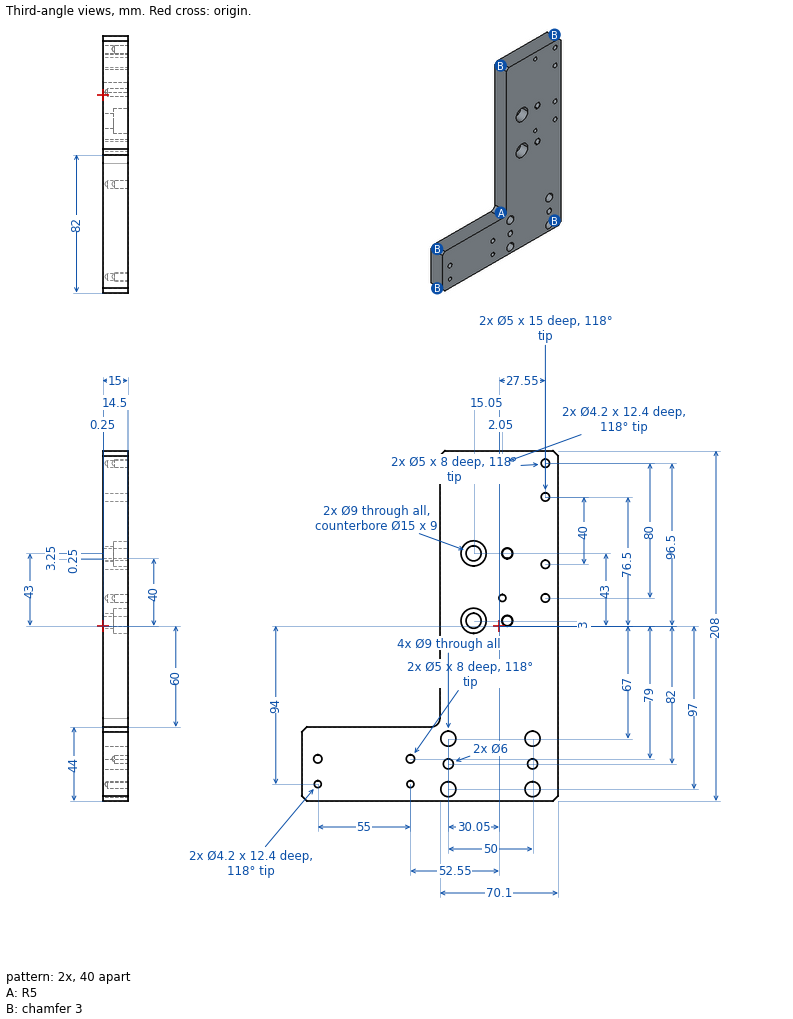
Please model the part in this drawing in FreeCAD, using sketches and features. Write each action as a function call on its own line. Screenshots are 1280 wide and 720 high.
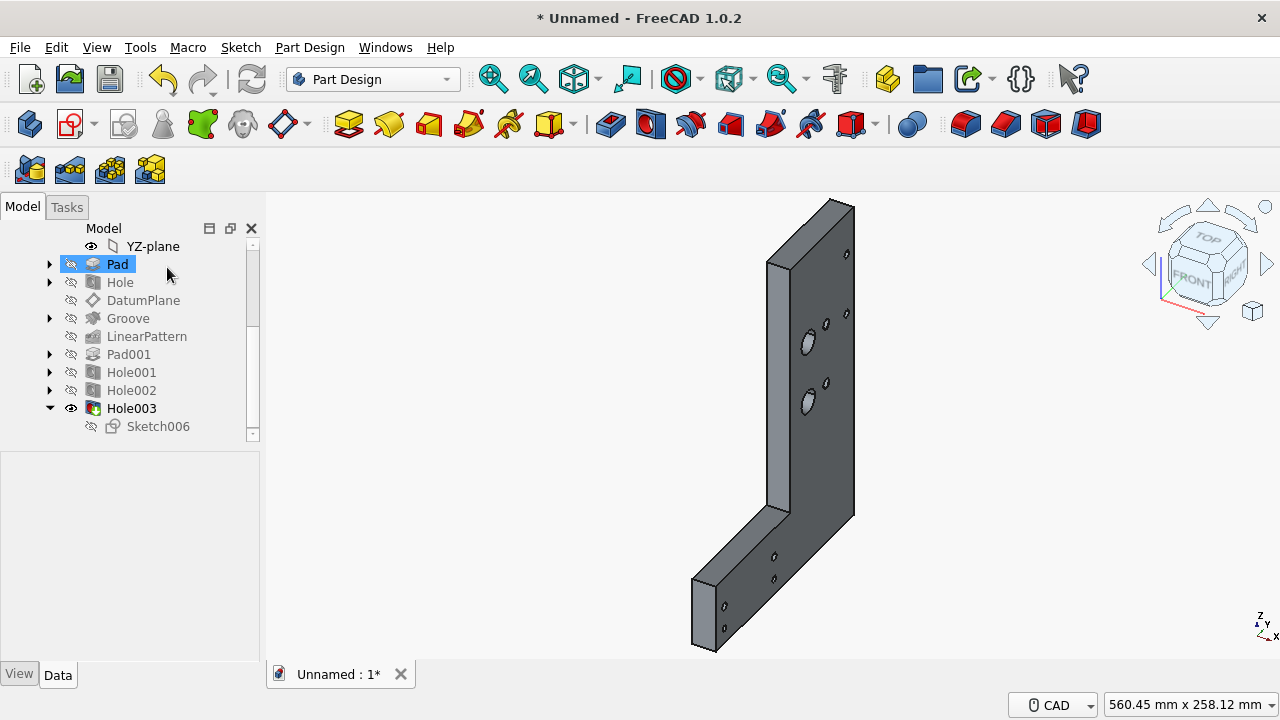
click(824, 477)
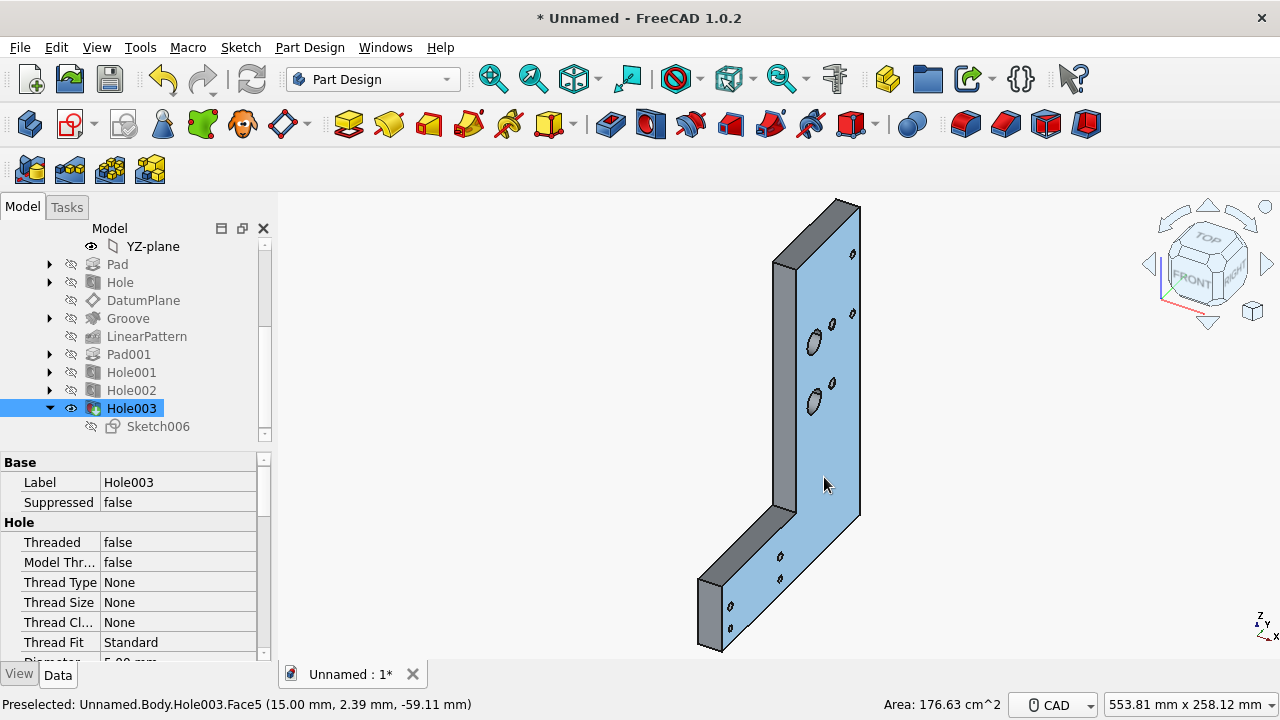
click(70, 124)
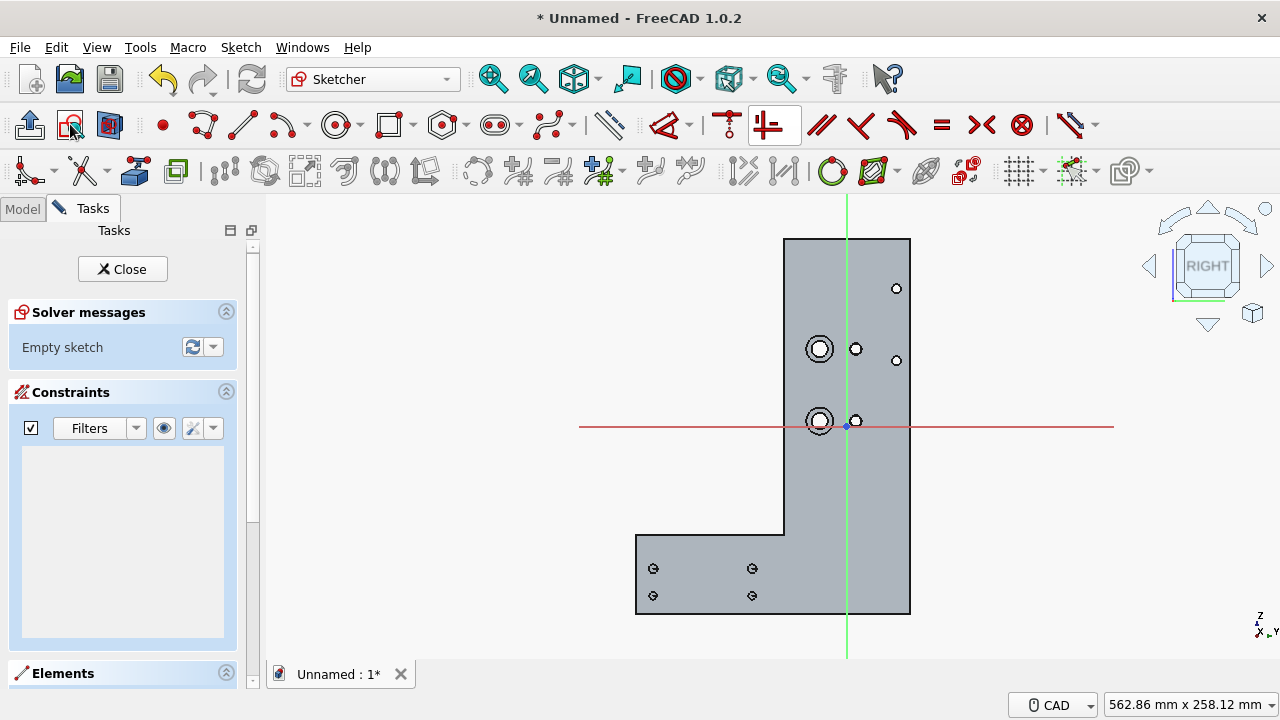
scroll(1115, 222, up, 2)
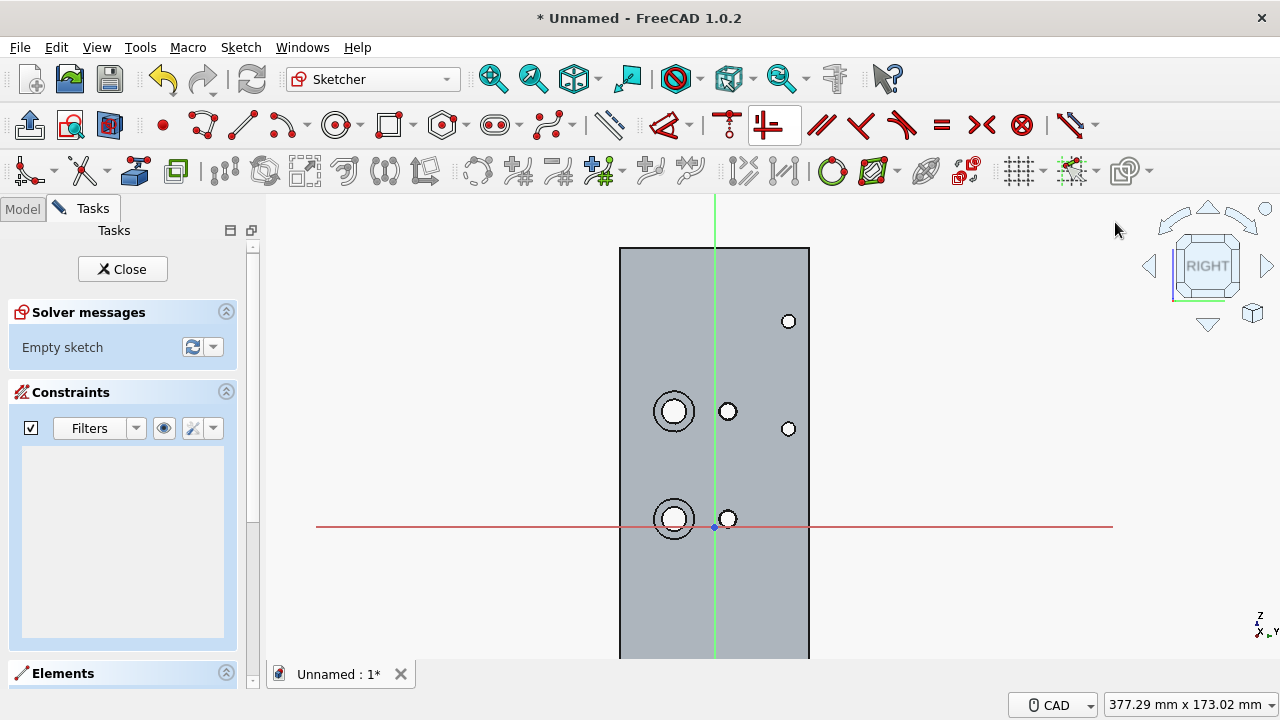
click(336, 126)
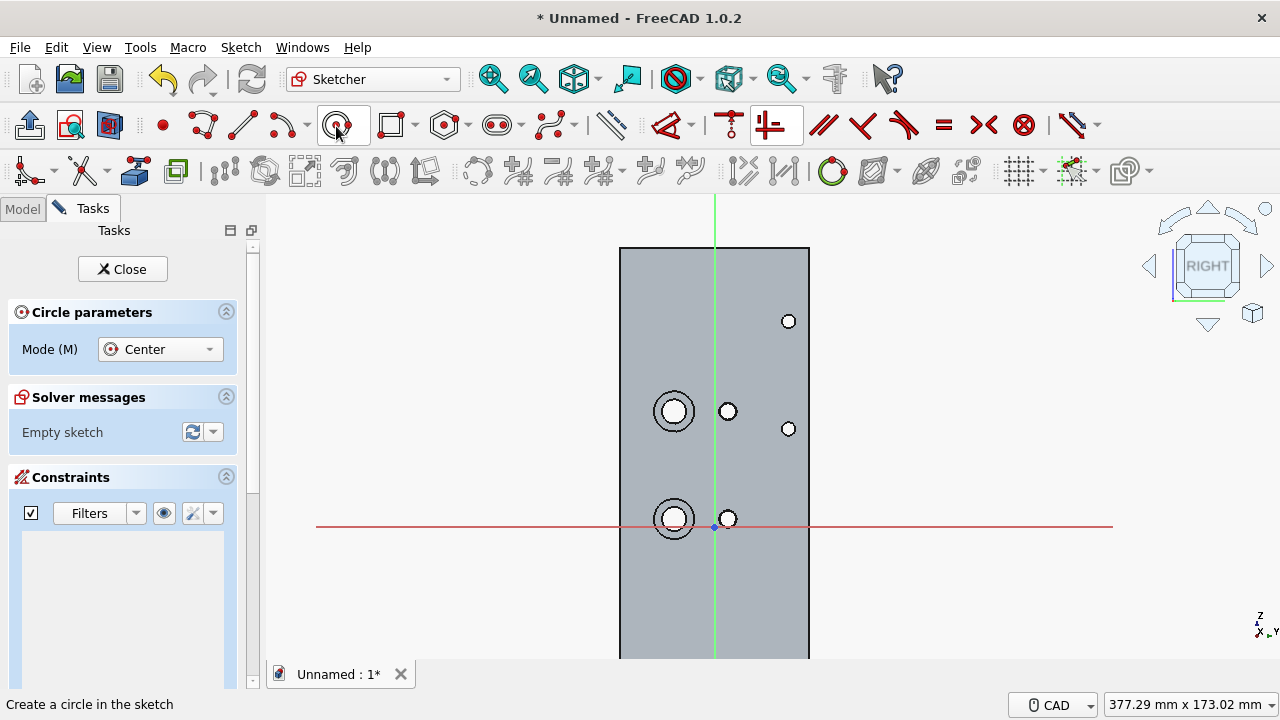
scroll(789, 268, up, 7)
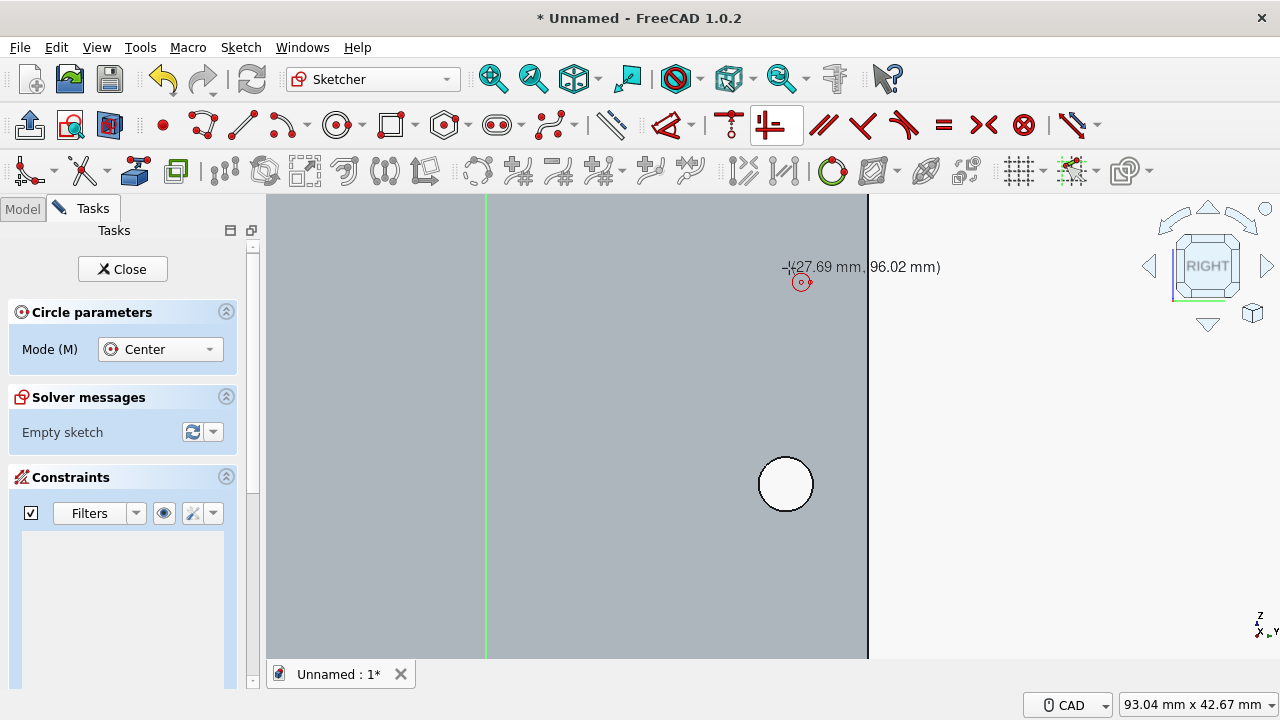
scroll(723, 311, down, 7)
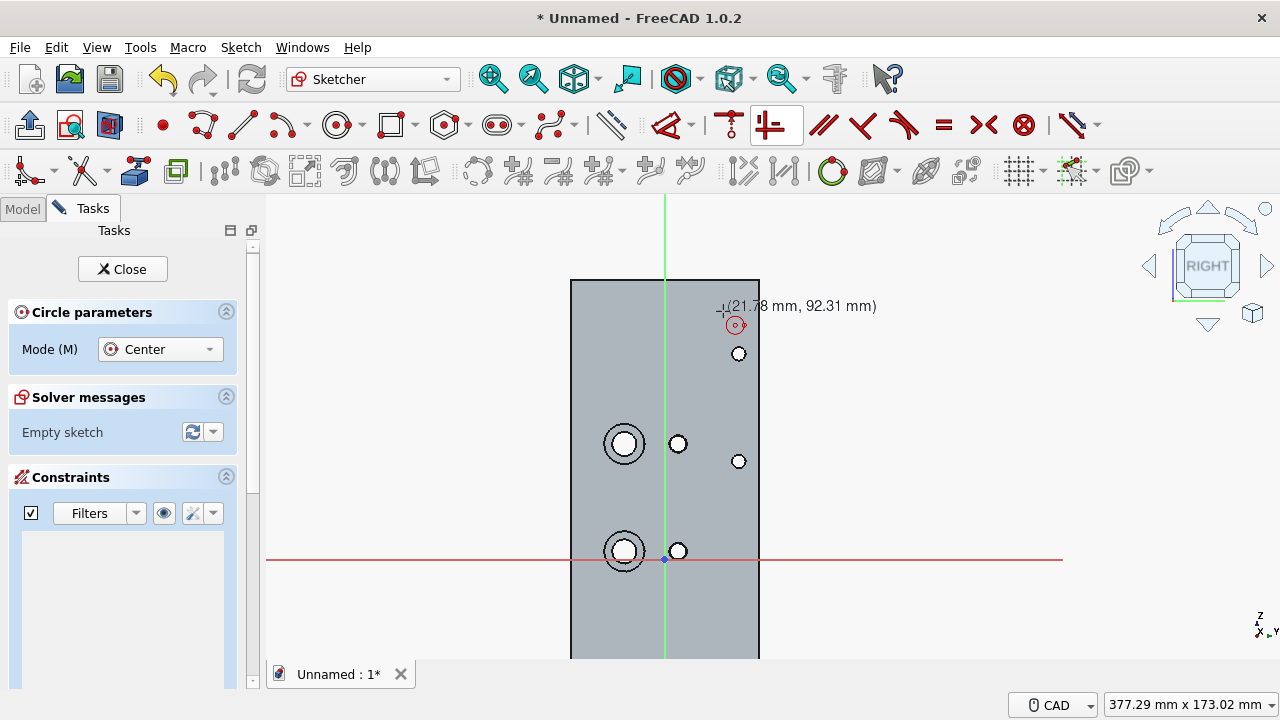
click(739, 300)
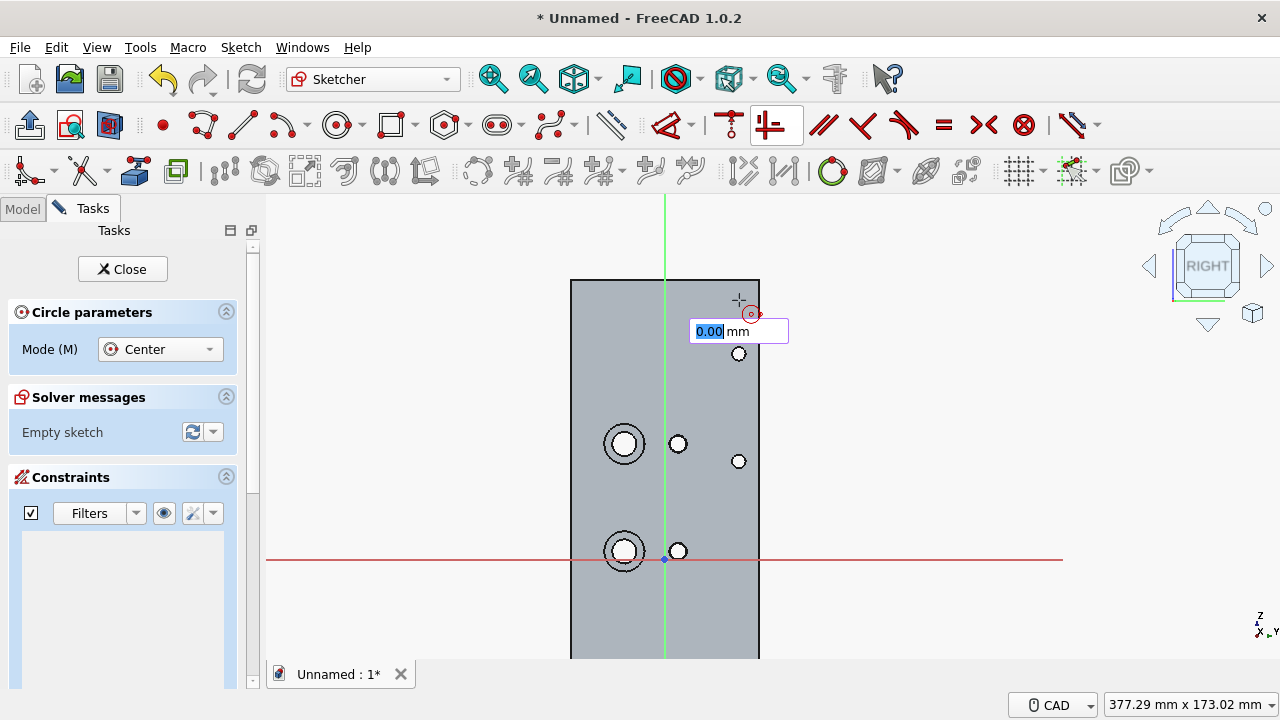
scroll(744, 295, up, 5)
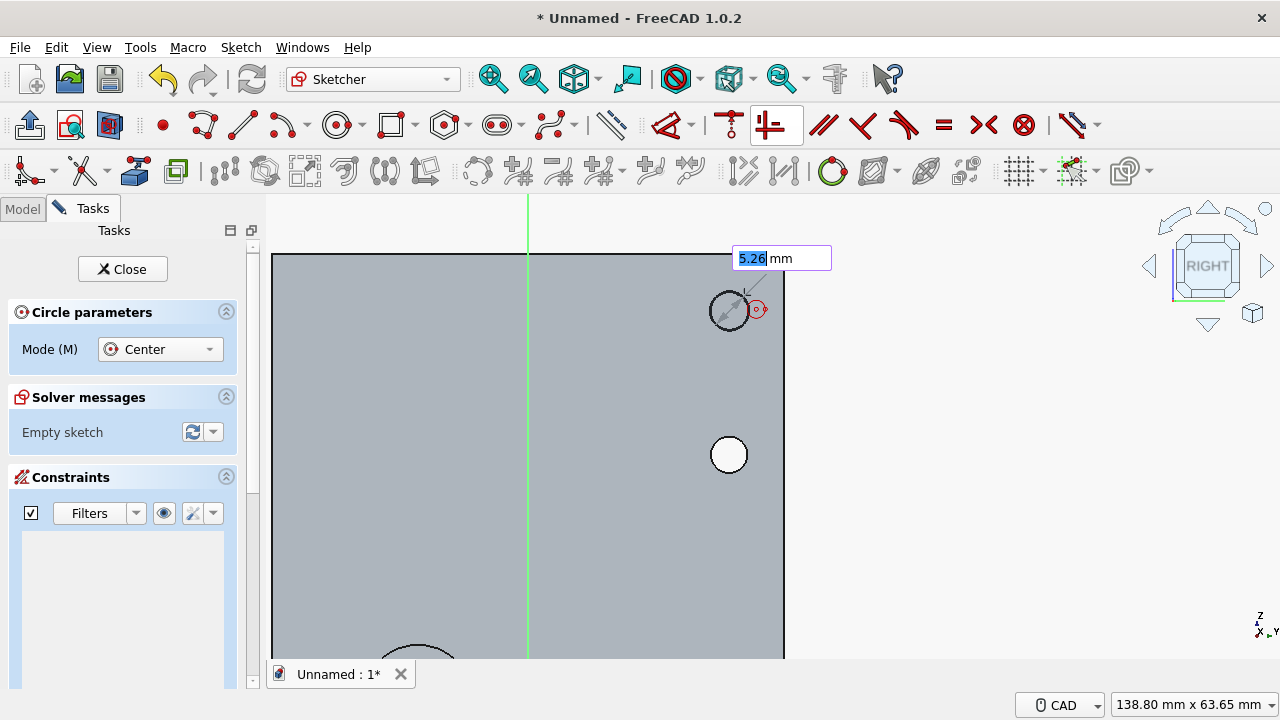
click(742, 296)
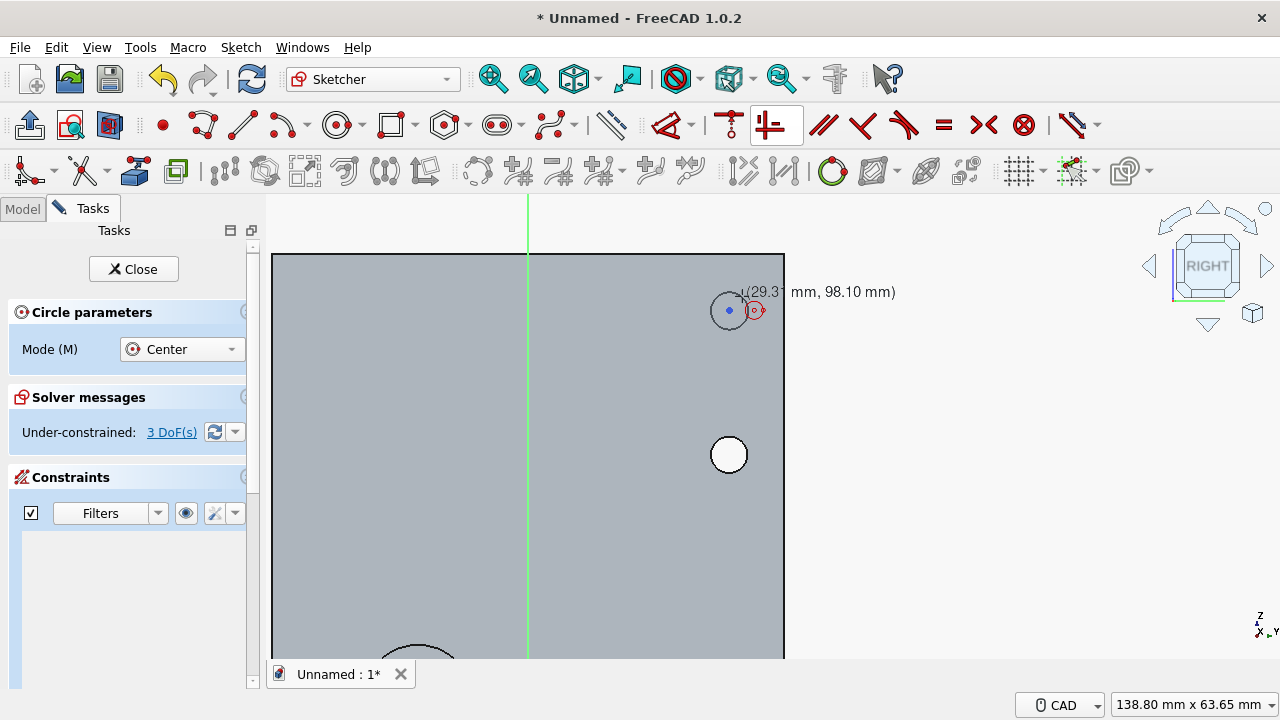
scroll(743, 295, down, 5)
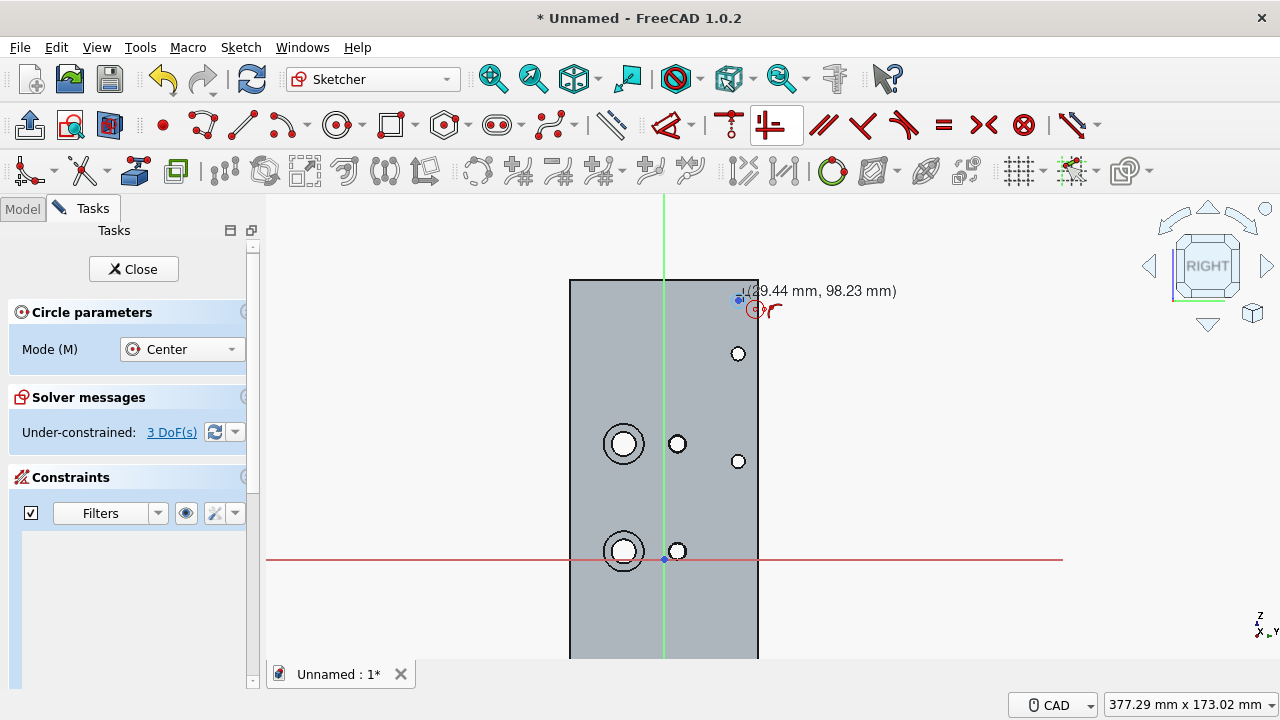
scroll(738, 515, up, 7)